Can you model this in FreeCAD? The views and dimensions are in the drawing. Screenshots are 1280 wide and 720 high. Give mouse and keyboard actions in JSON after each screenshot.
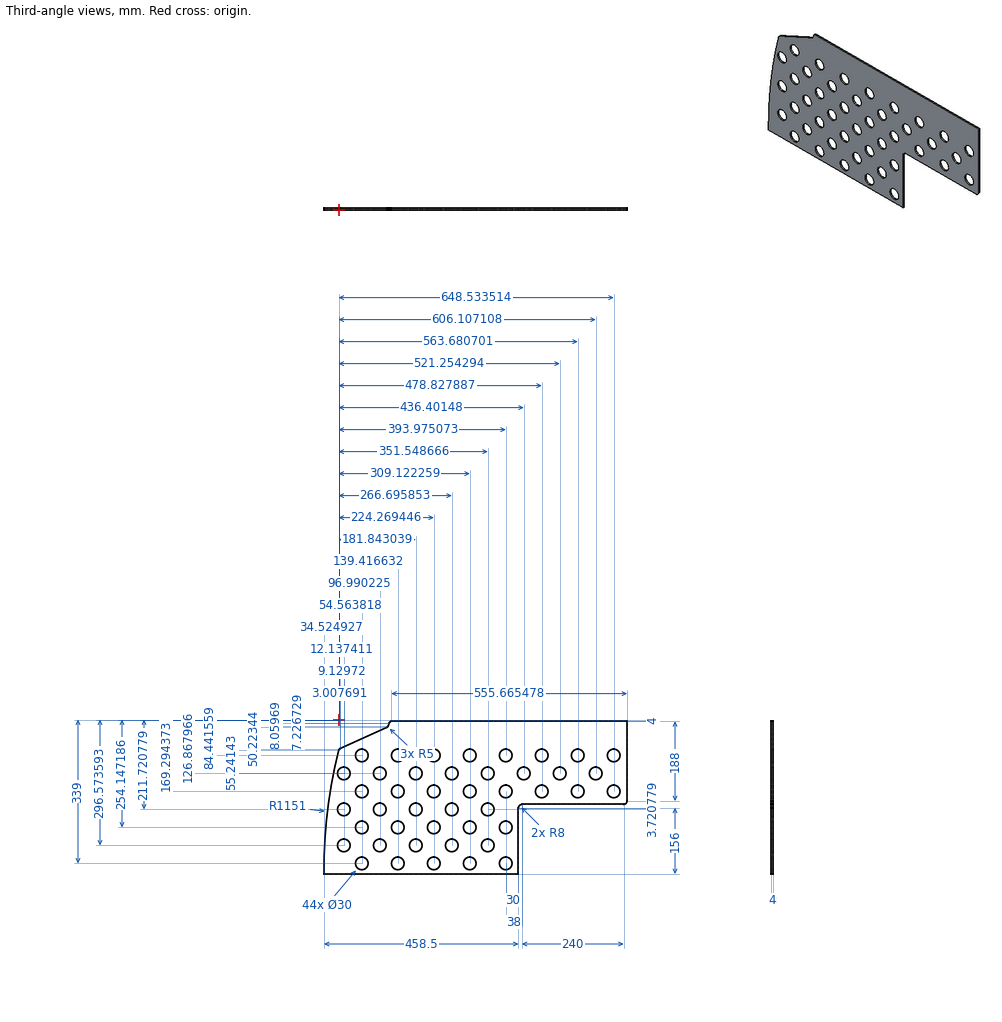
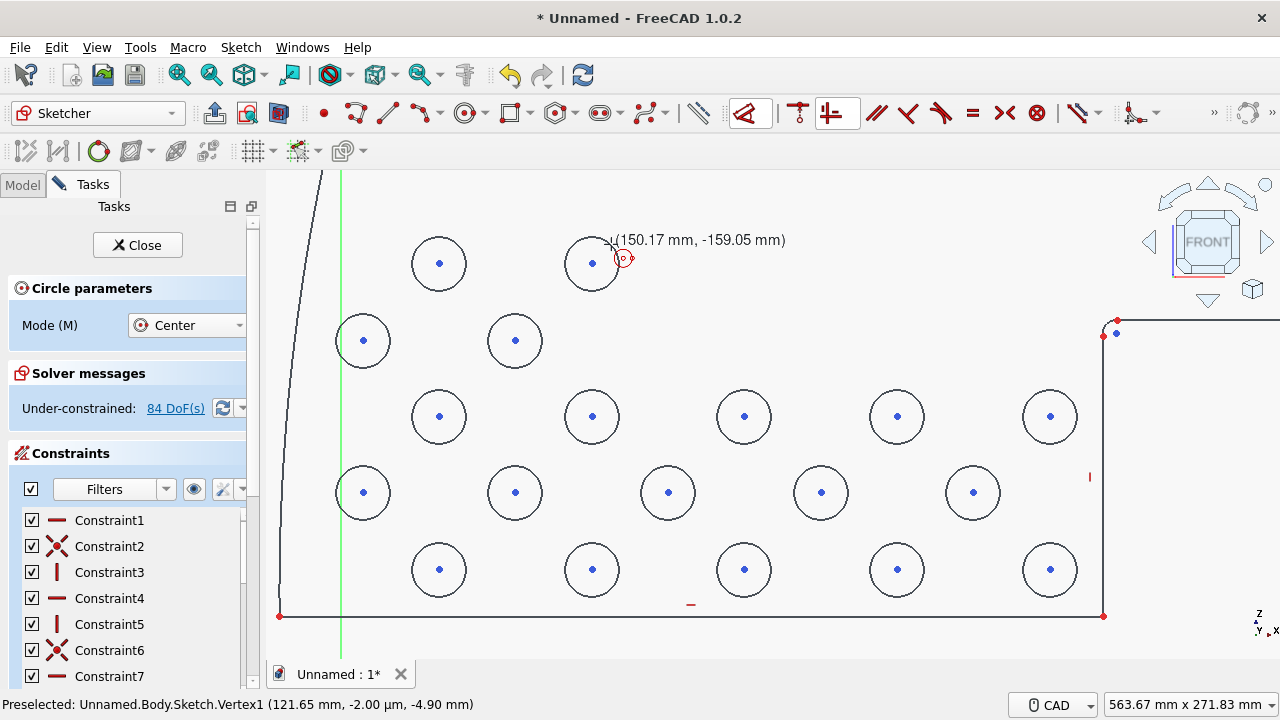
{"action": "left_click", "coordinate": [668, 340]}
{"action": "left_click", "coordinate": [687, 321]}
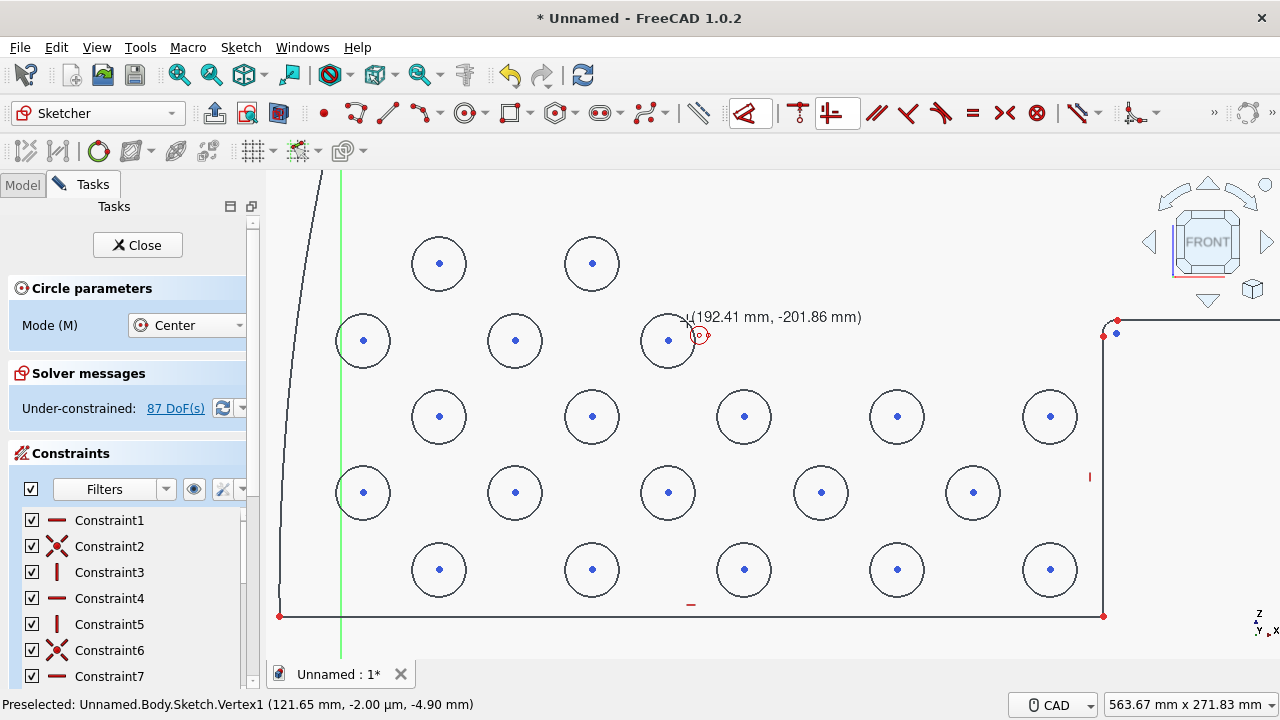
{"action": "left_click", "coordinate": [821, 340]}
{"action": "left_click", "coordinate": [840, 321]}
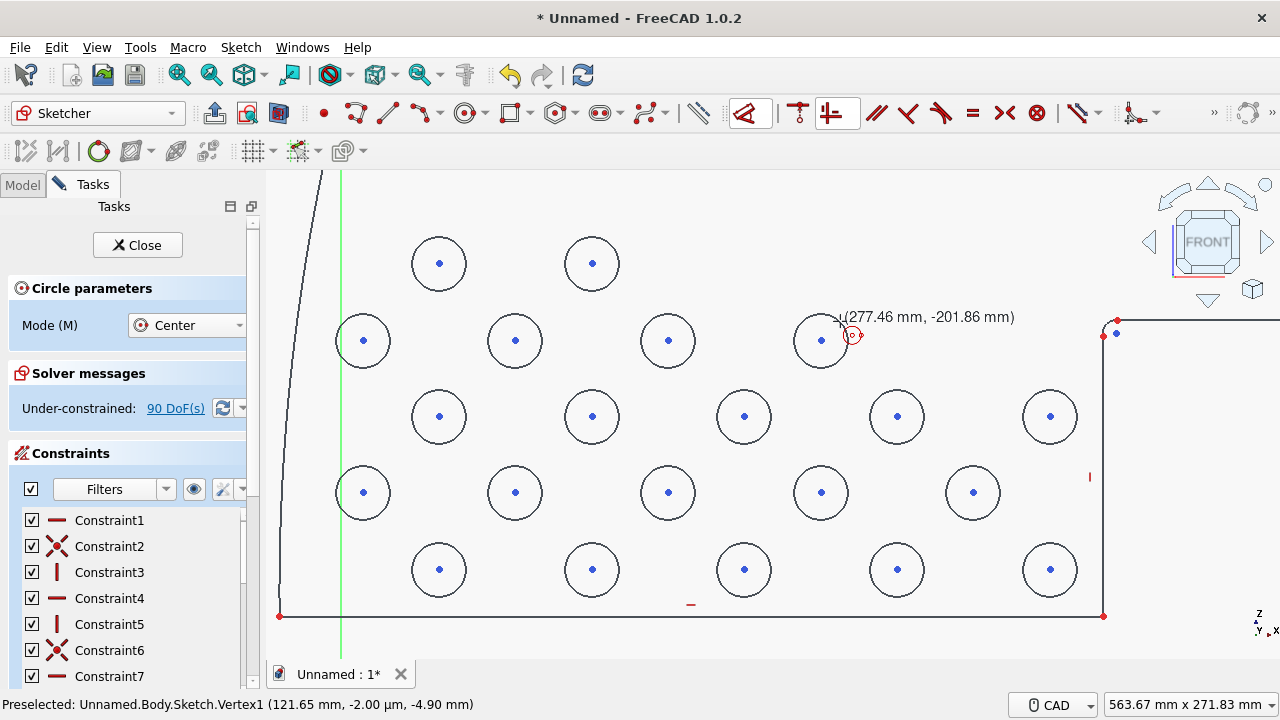
{"action": "left_click", "coordinate": [744, 263]}
{"action": "left_click", "coordinate": [763, 244]}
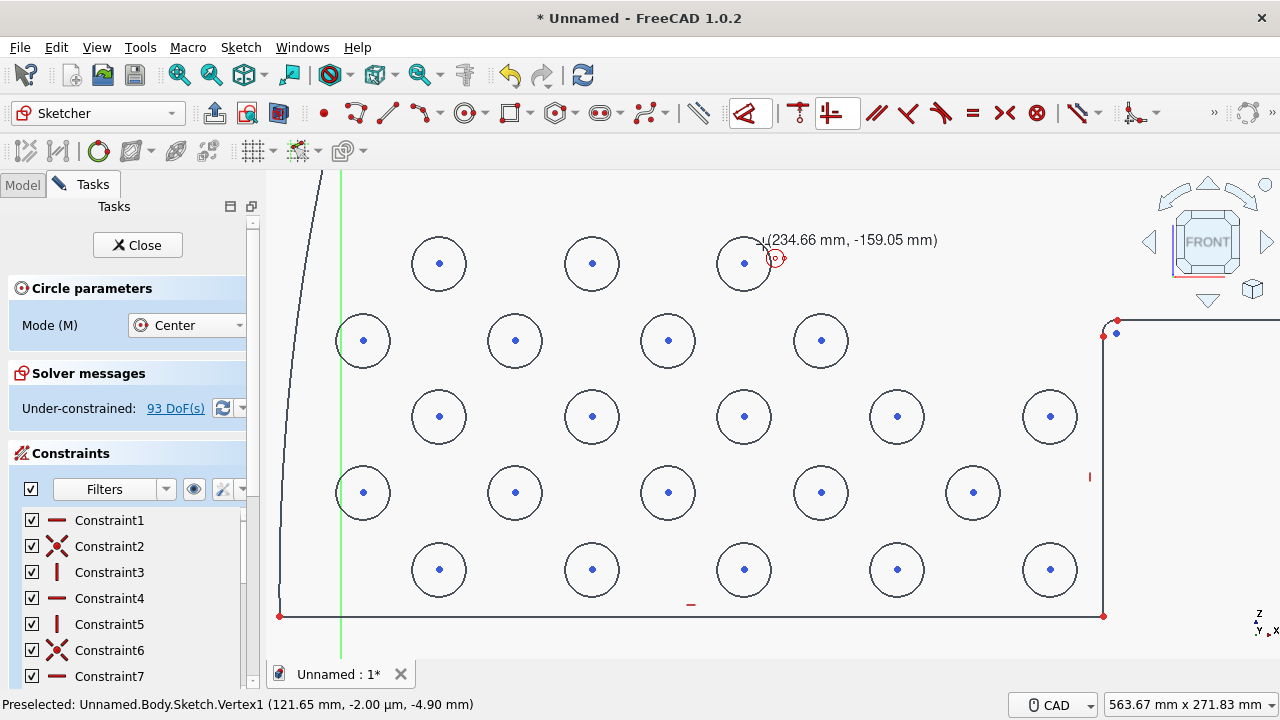
{"action": "left_click", "coordinate": [897, 263]}
{"action": "left_click", "coordinate": [916, 244]}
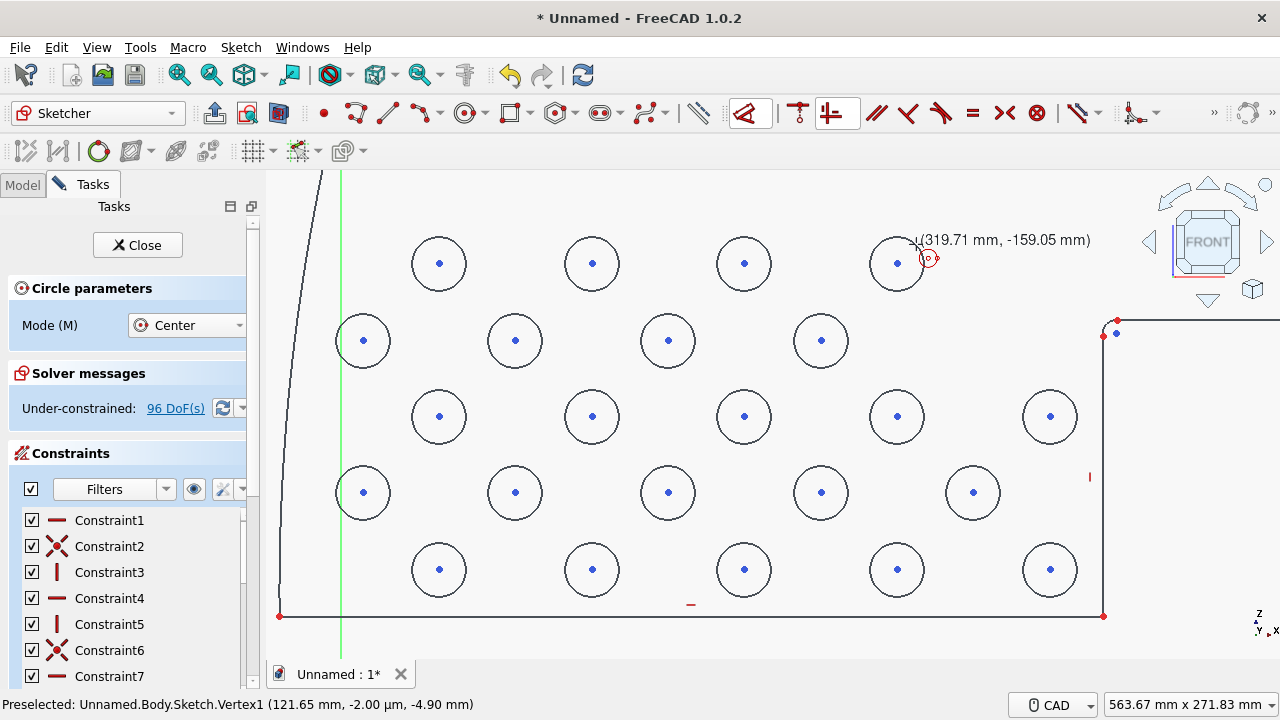
{"action": "scroll", "coordinate": [527, 519], "scroll_direction": "down", "scroll_amount": 4}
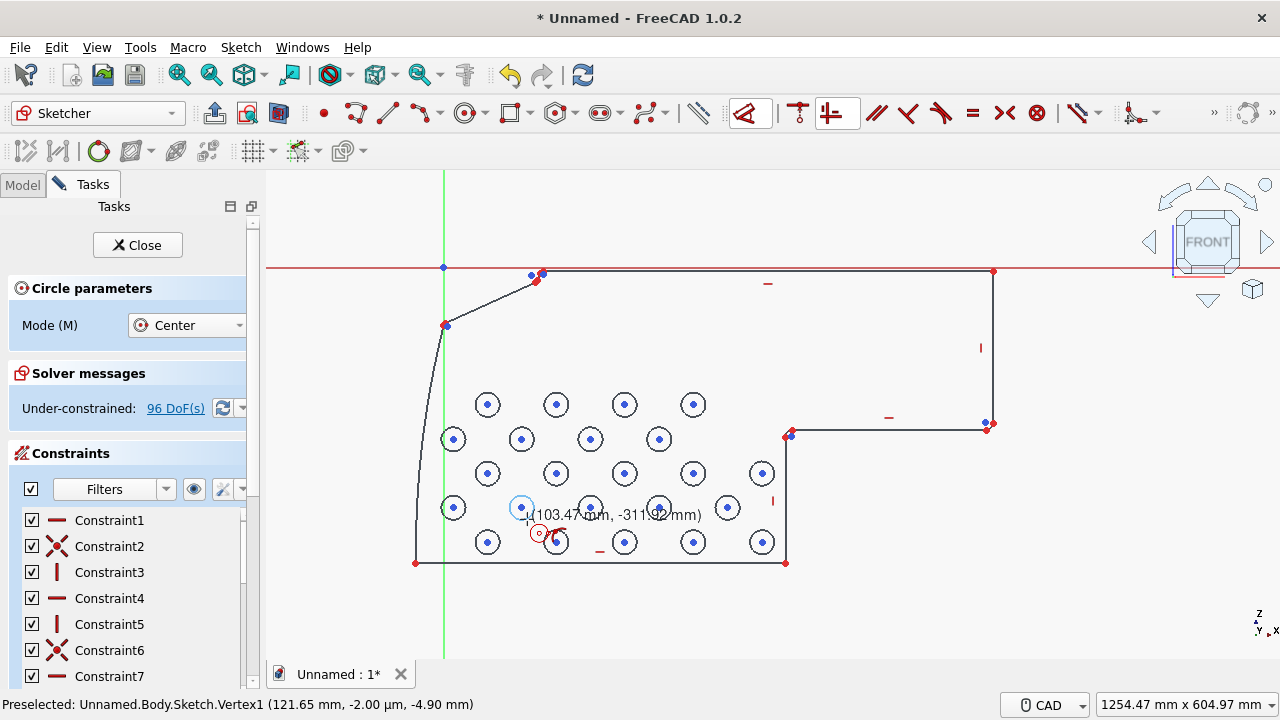
{"action": "scroll", "coordinate": [453, 370], "scroll_direction": "up", "scroll_amount": 4}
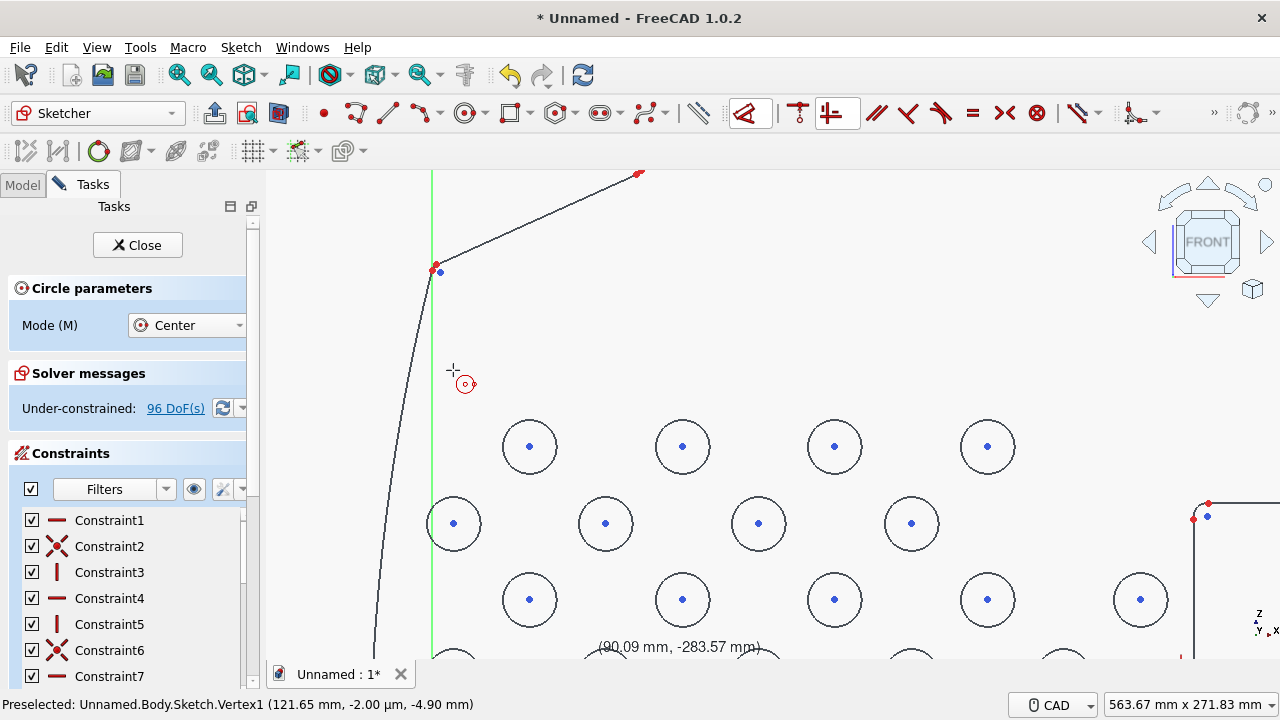
{"action": "left_click", "coordinate": [453, 370]}
{"action": "left_click", "coordinate": [473, 351]}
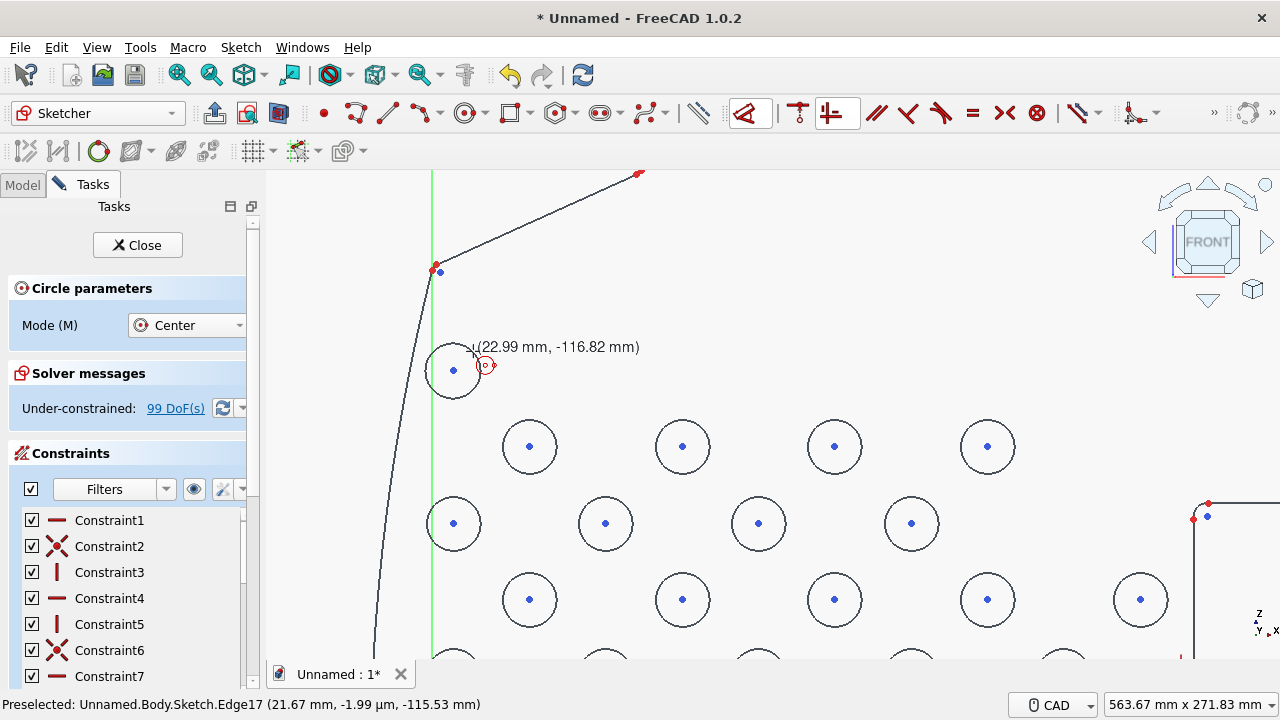
{"action": "left_click", "coordinate": [606, 370]}
{"action": "left_click", "coordinate": [625, 351]}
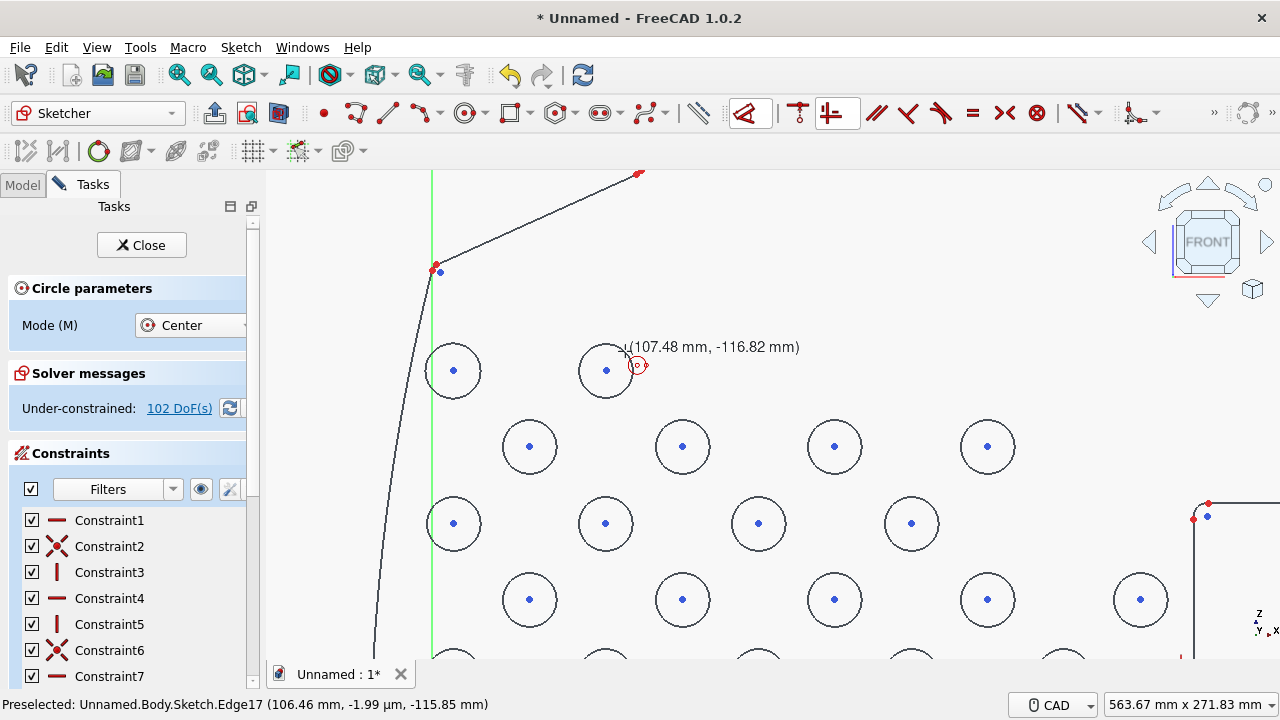
{"action": "left_click", "coordinate": [530, 294]}
{"action": "left_click", "coordinate": [549, 275]}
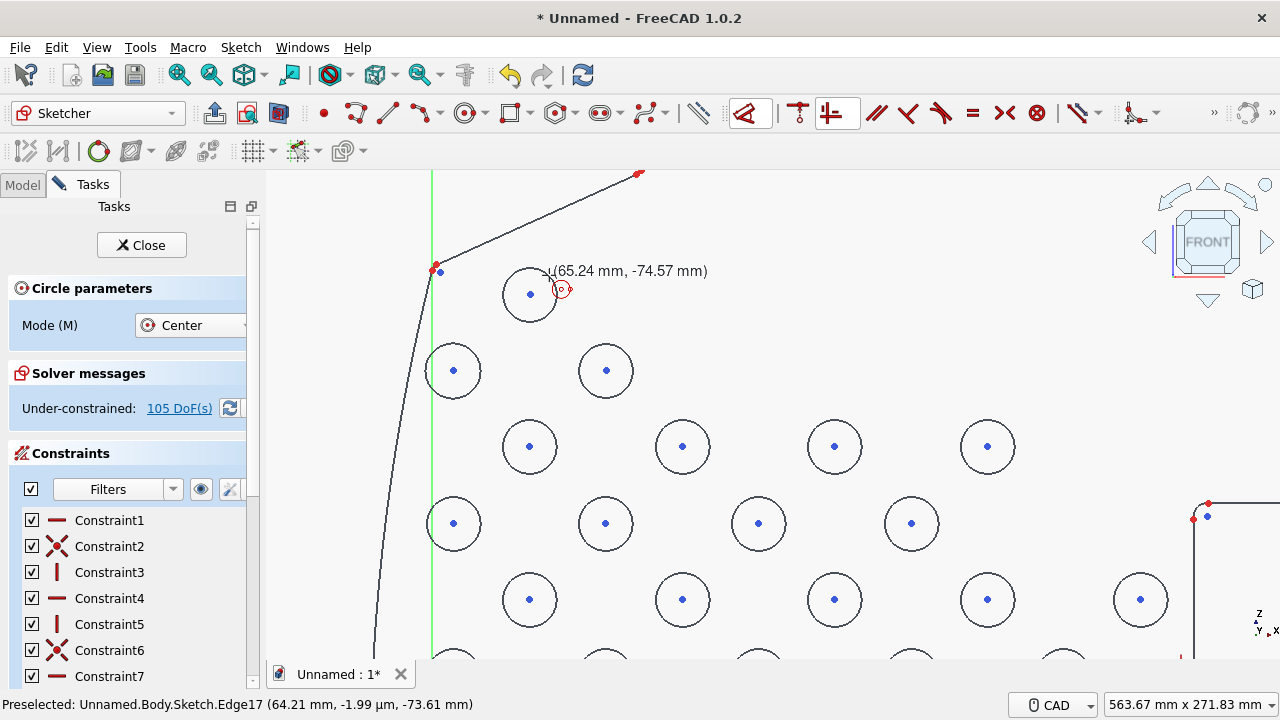
{"action": "left_click", "coordinate": [682, 294]}
{"action": "left_click", "coordinate": [702, 275]}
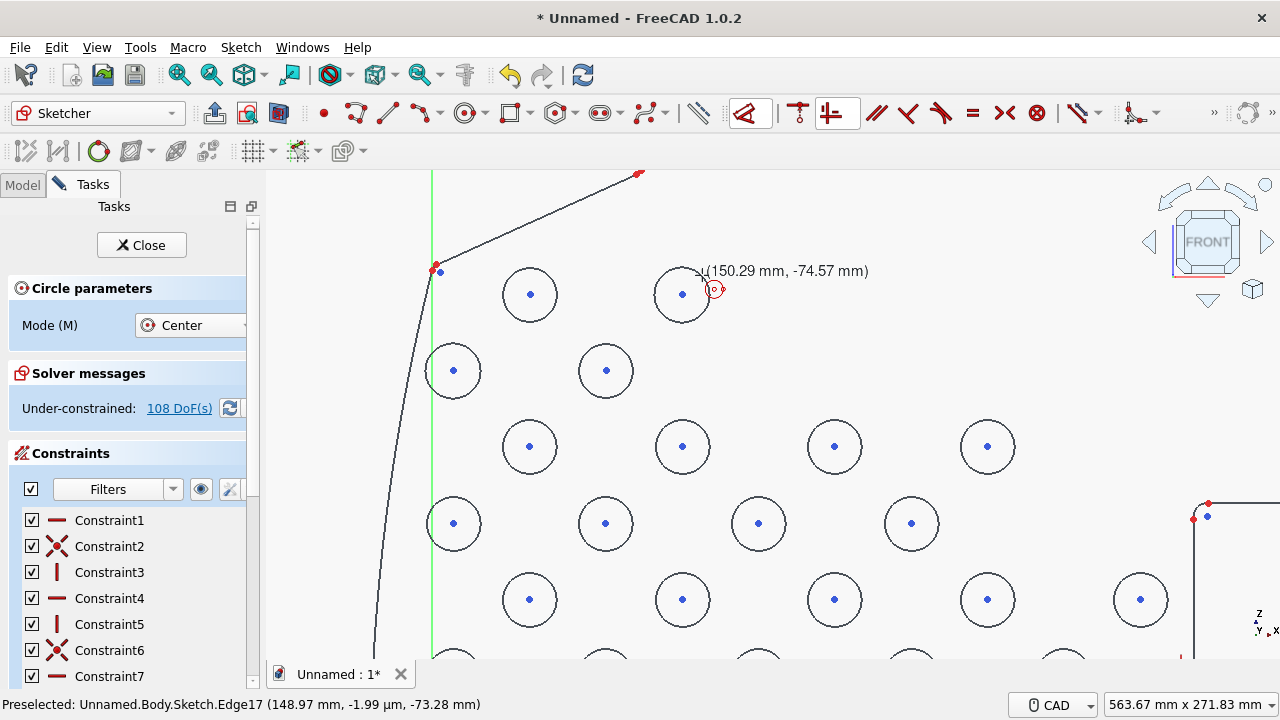
{"action": "left_click", "coordinate": [759, 370]}
{"action": "left_click", "coordinate": [778, 351]}